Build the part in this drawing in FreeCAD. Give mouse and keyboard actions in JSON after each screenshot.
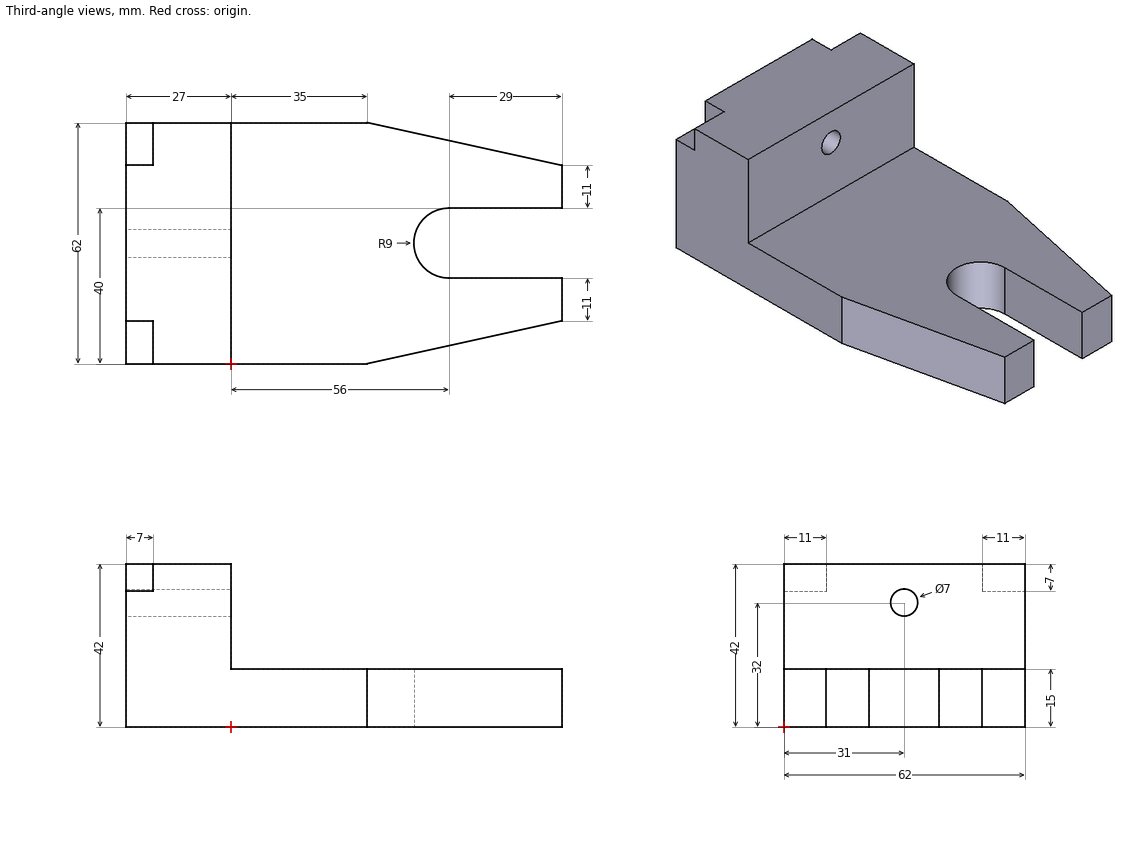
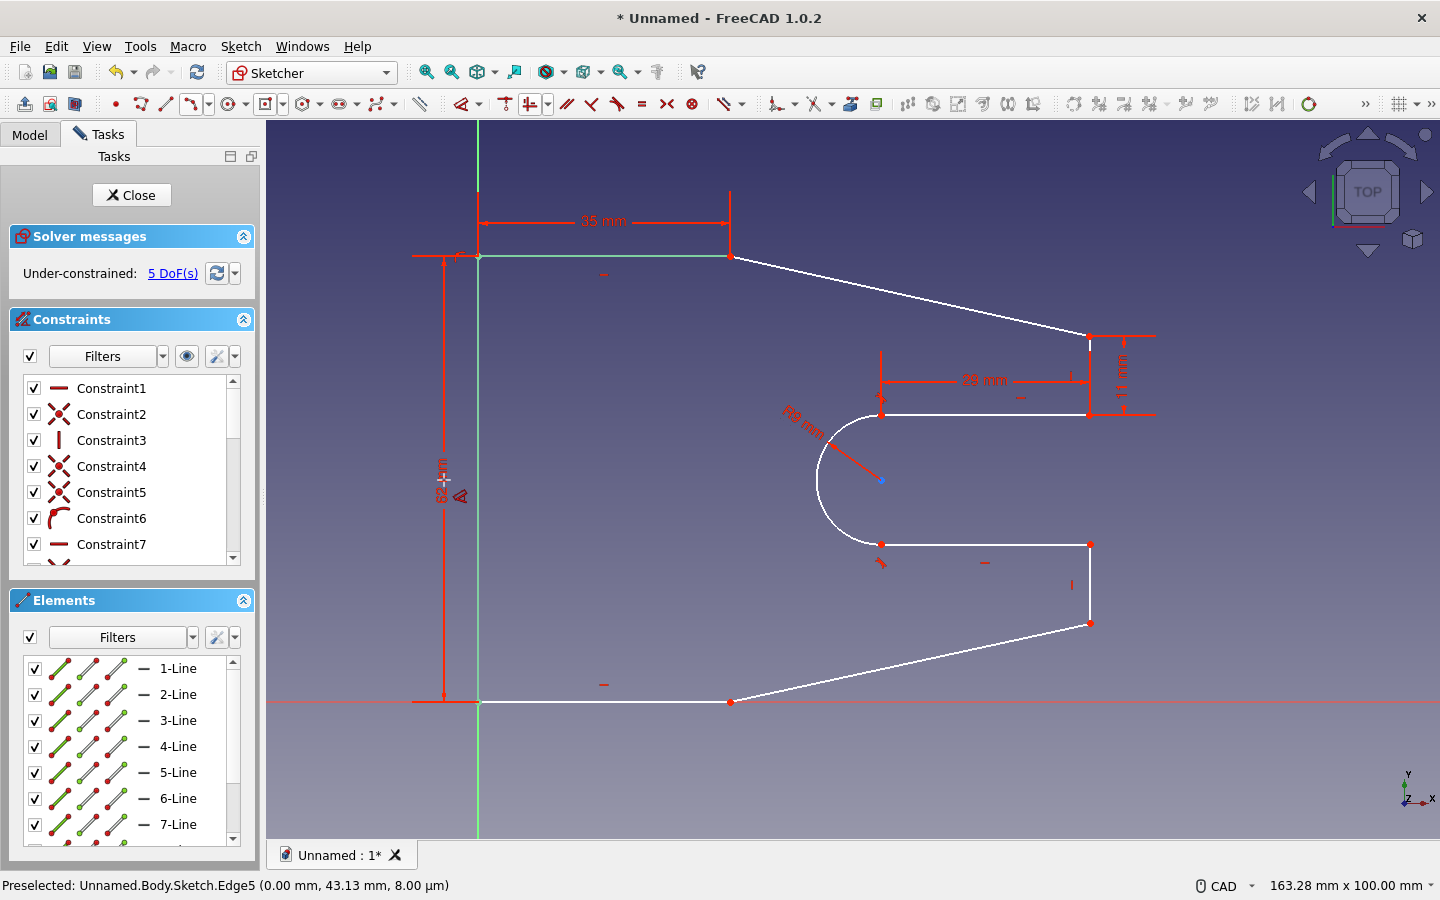
{"action": "left_click", "coordinate": [554, 702]}
{"action": "left_click", "coordinate": [604, 736]}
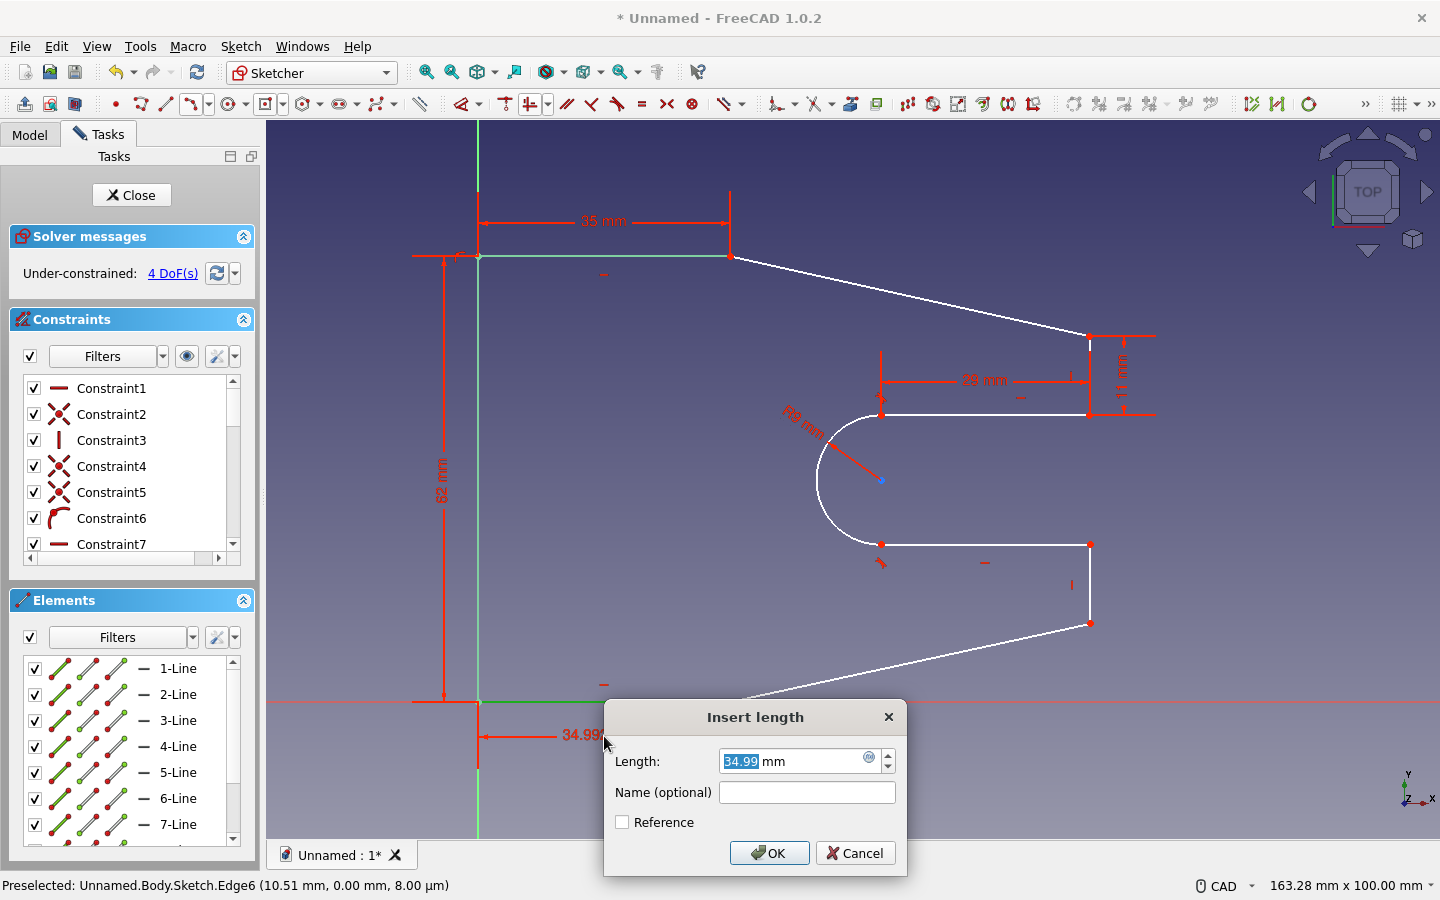
{"action": "type", "text": "35"}
{"action": "key", "text": "Return"}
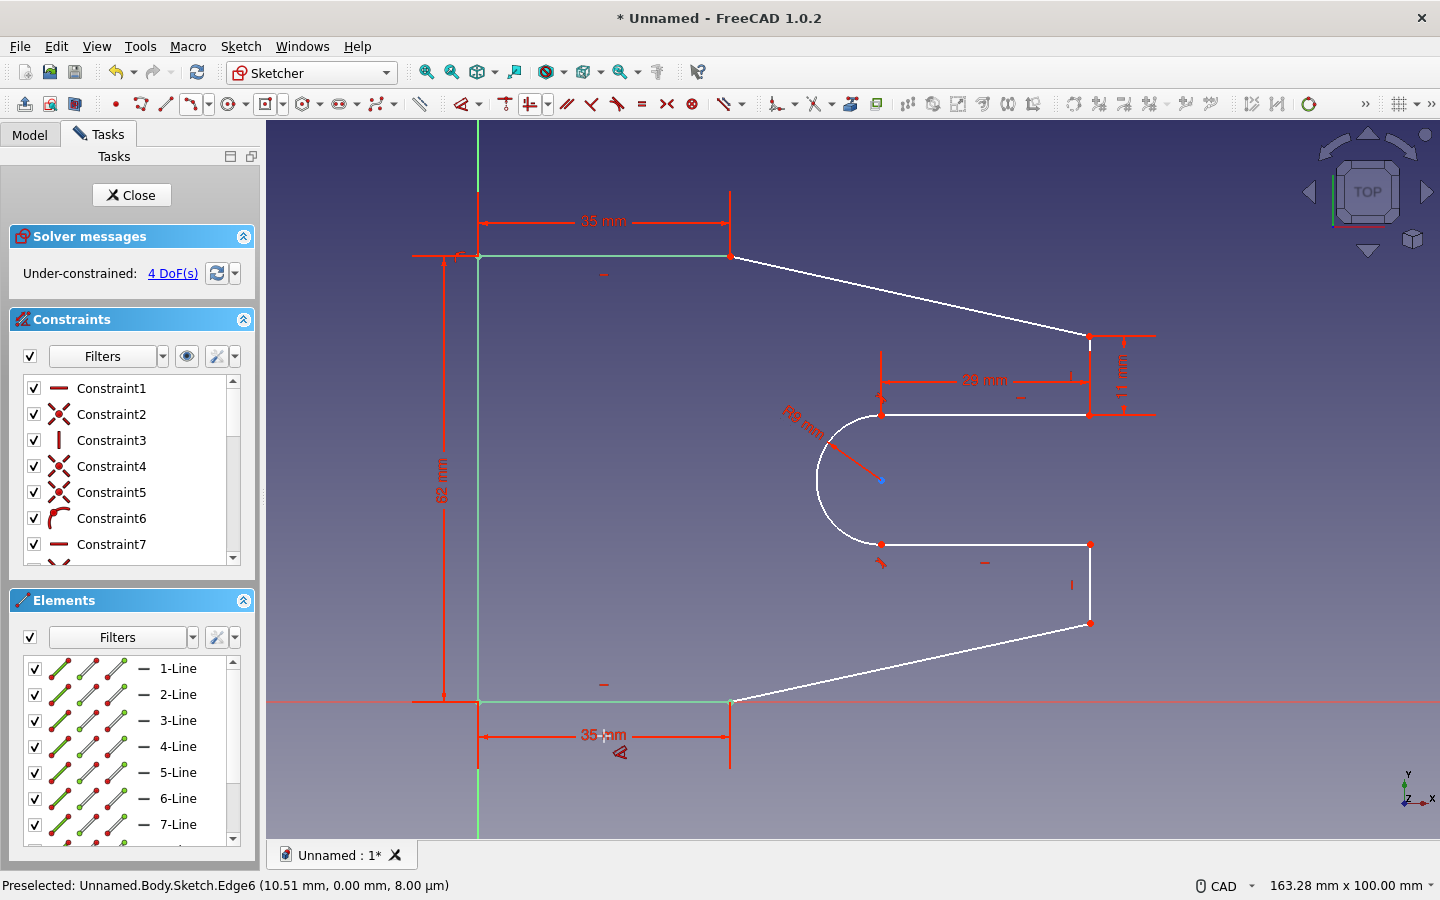
{"action": "left_click", "coordinate": [1090, 600]}
{"action": "left_click", "coordinate": [1124, 584]}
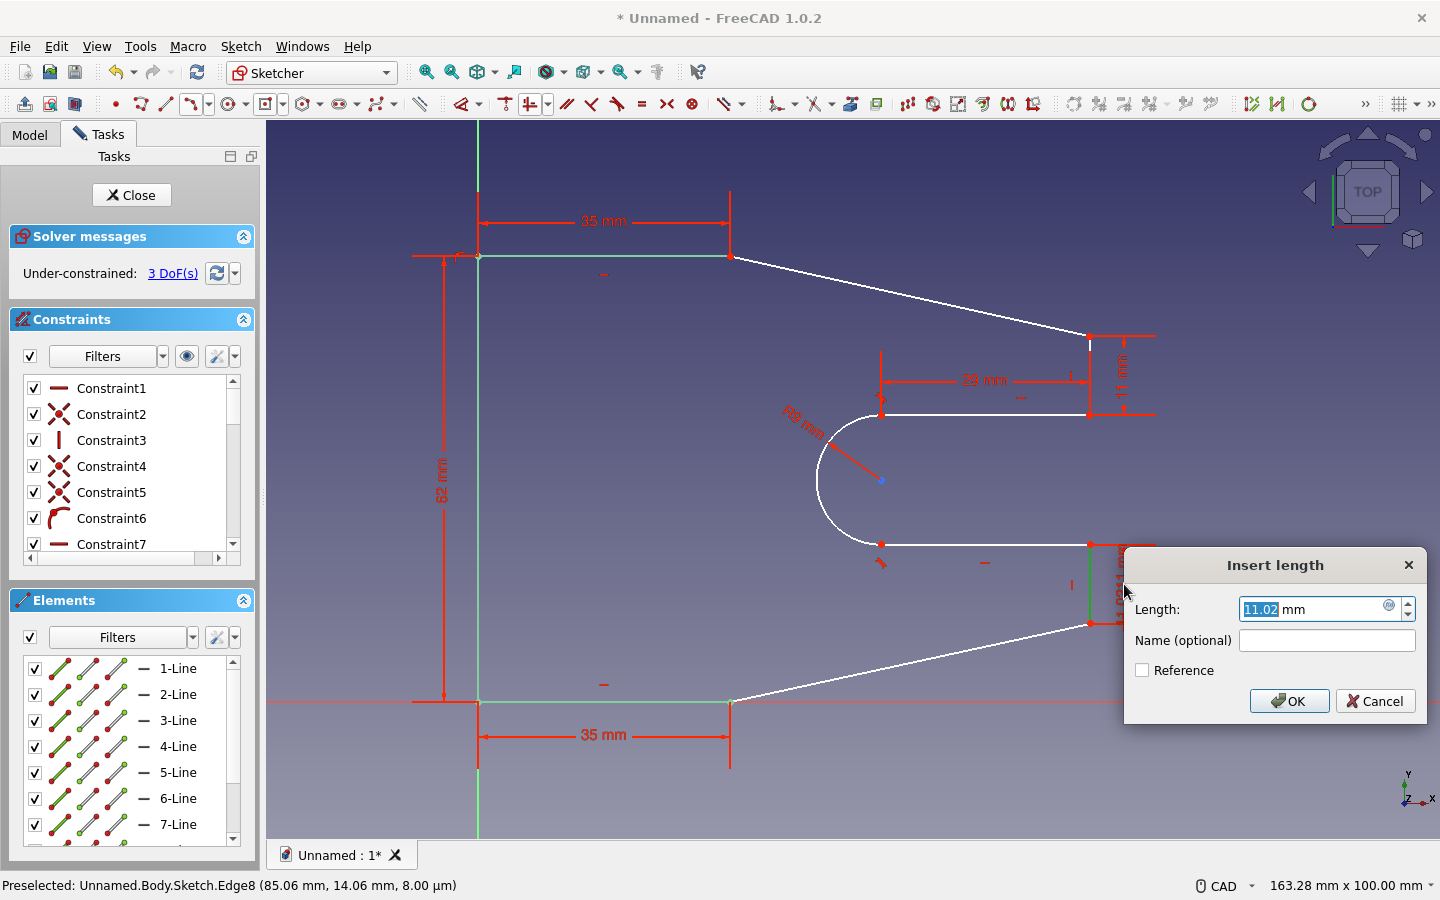
{"action": "type", "text": "11"}
{"action": "key", "text": "Return"}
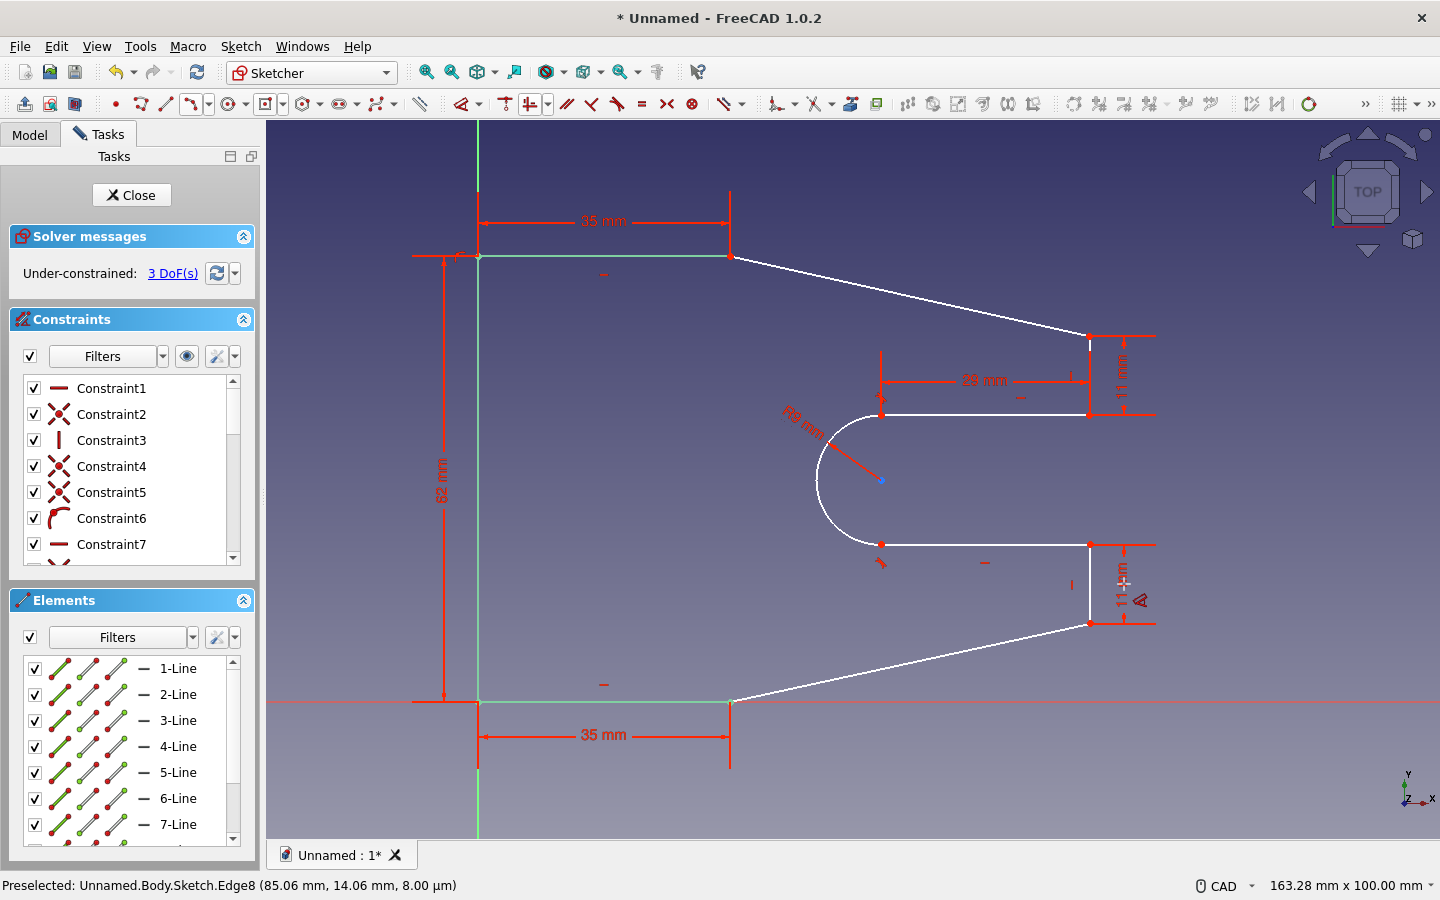
{"action": "left_click", "coordinate": [1027, 545]}
{"action": "left_click", "coordinate": [986, 579]}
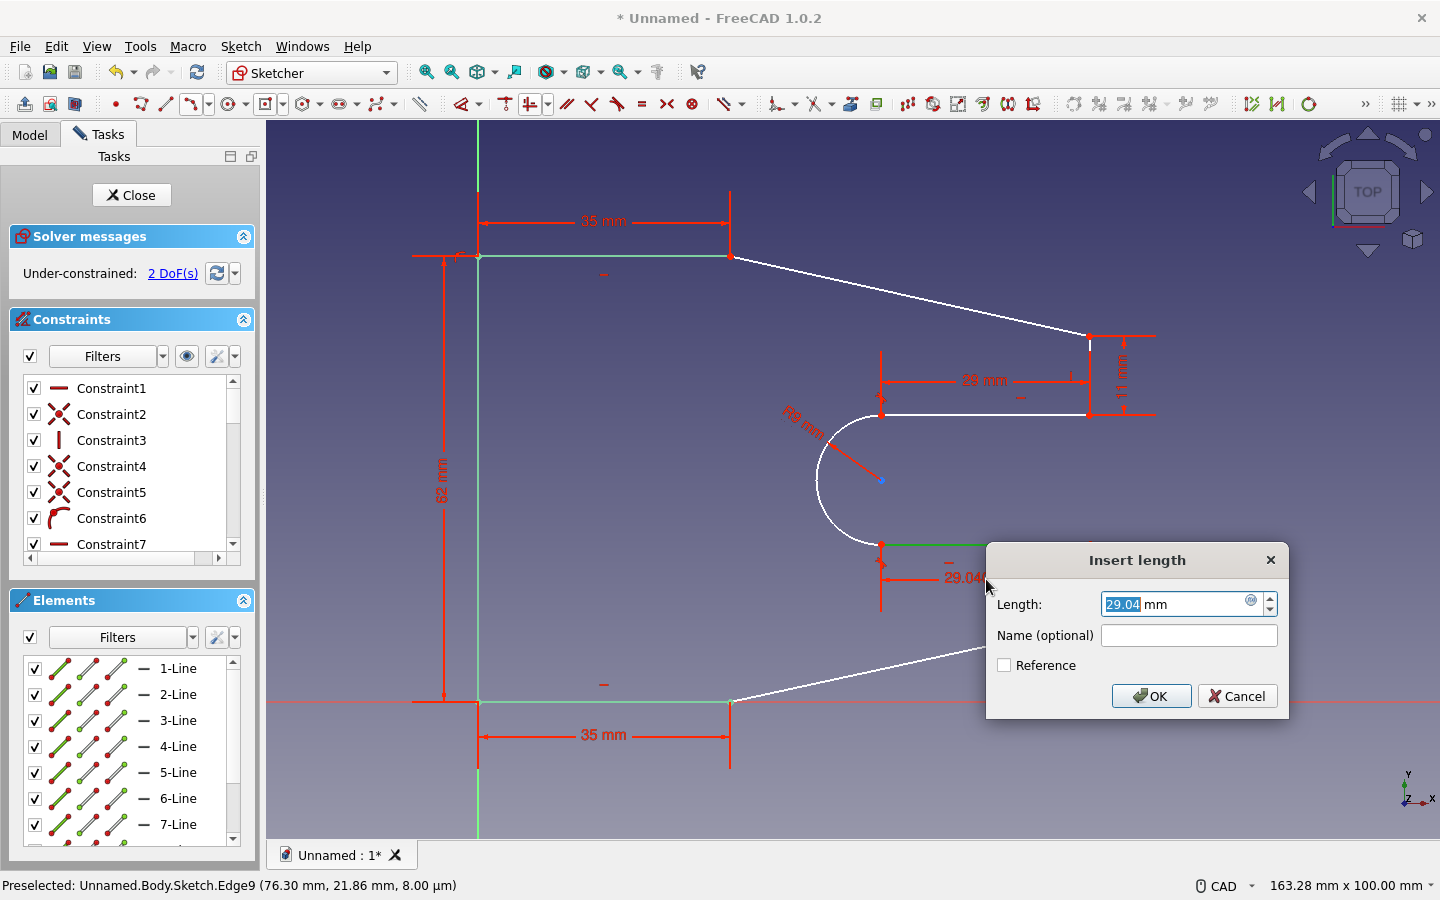
{"action": "type", "text": "29"}
{"action": "key", "text": "Return"}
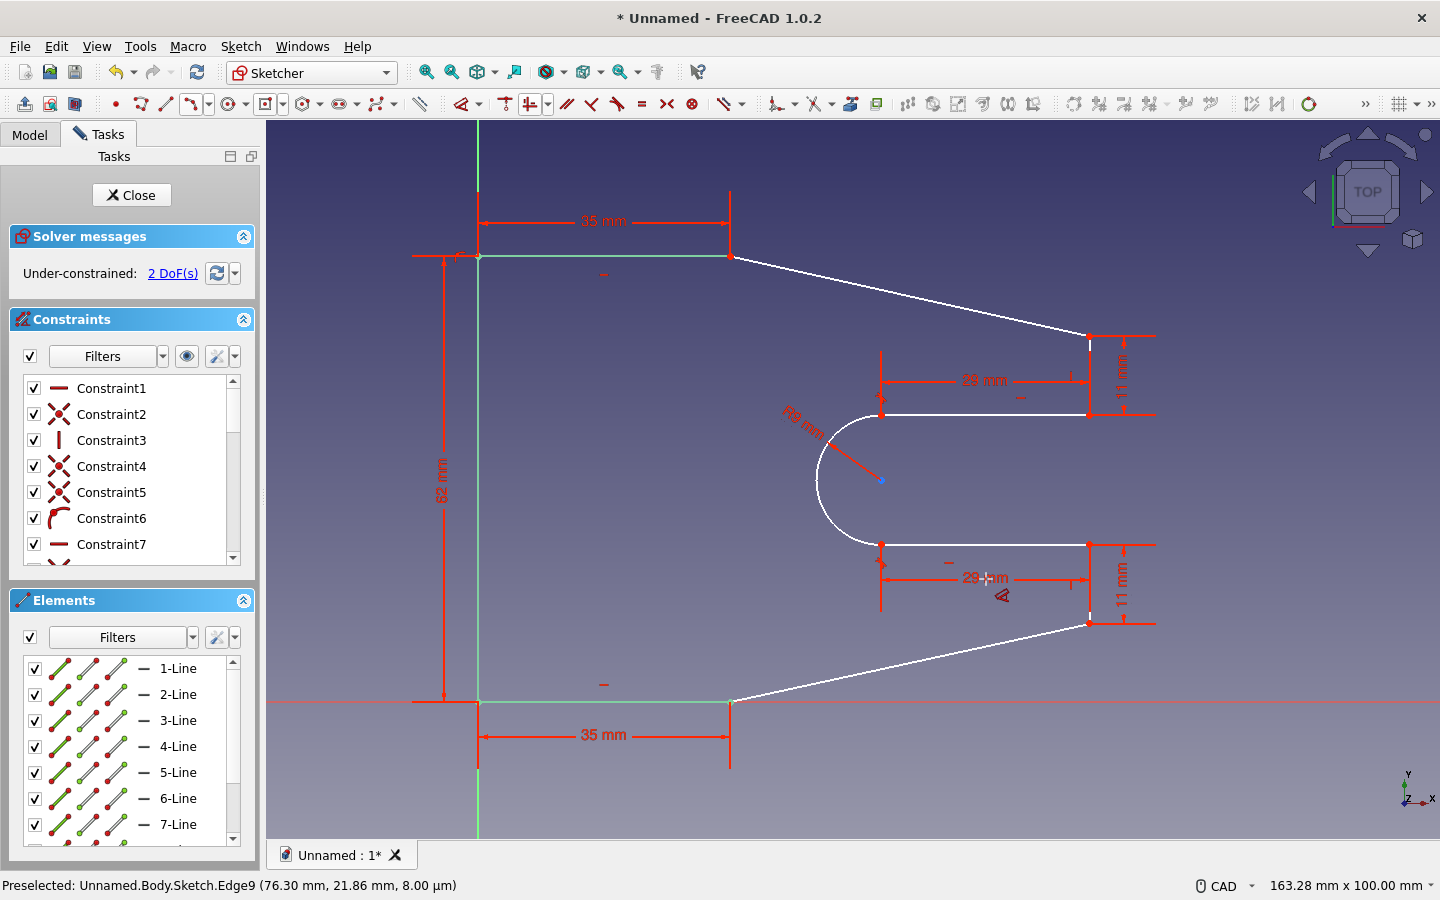
{"action": "left_click", "coordinate": [881, 415]}
{"action": "left_click", "coordinate": [680, 736]}